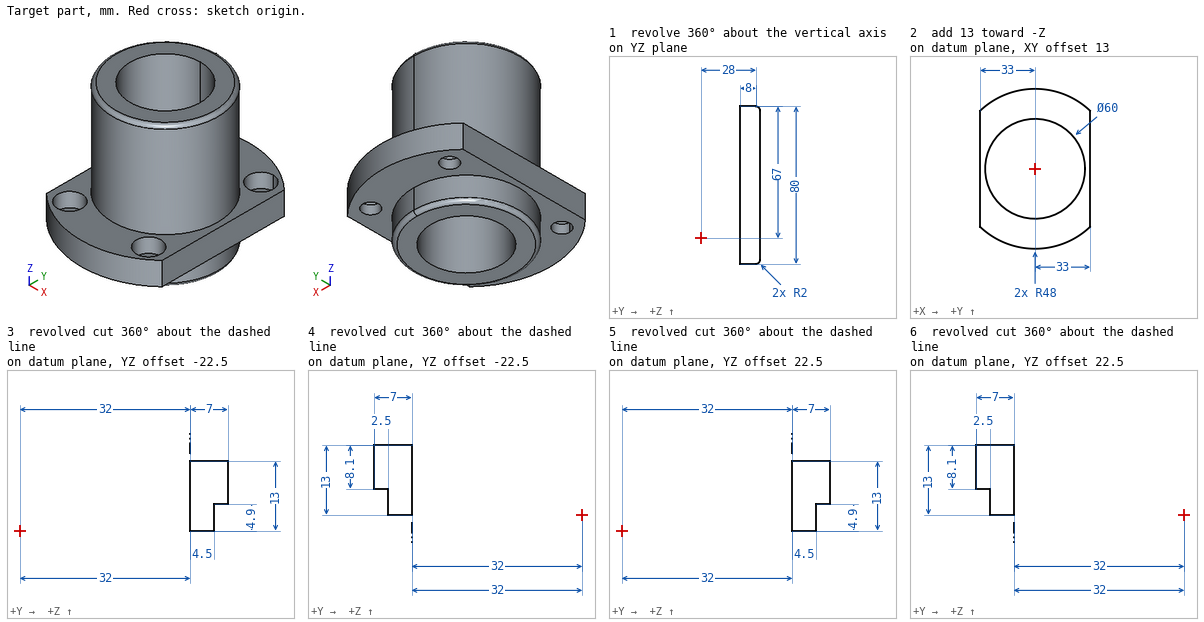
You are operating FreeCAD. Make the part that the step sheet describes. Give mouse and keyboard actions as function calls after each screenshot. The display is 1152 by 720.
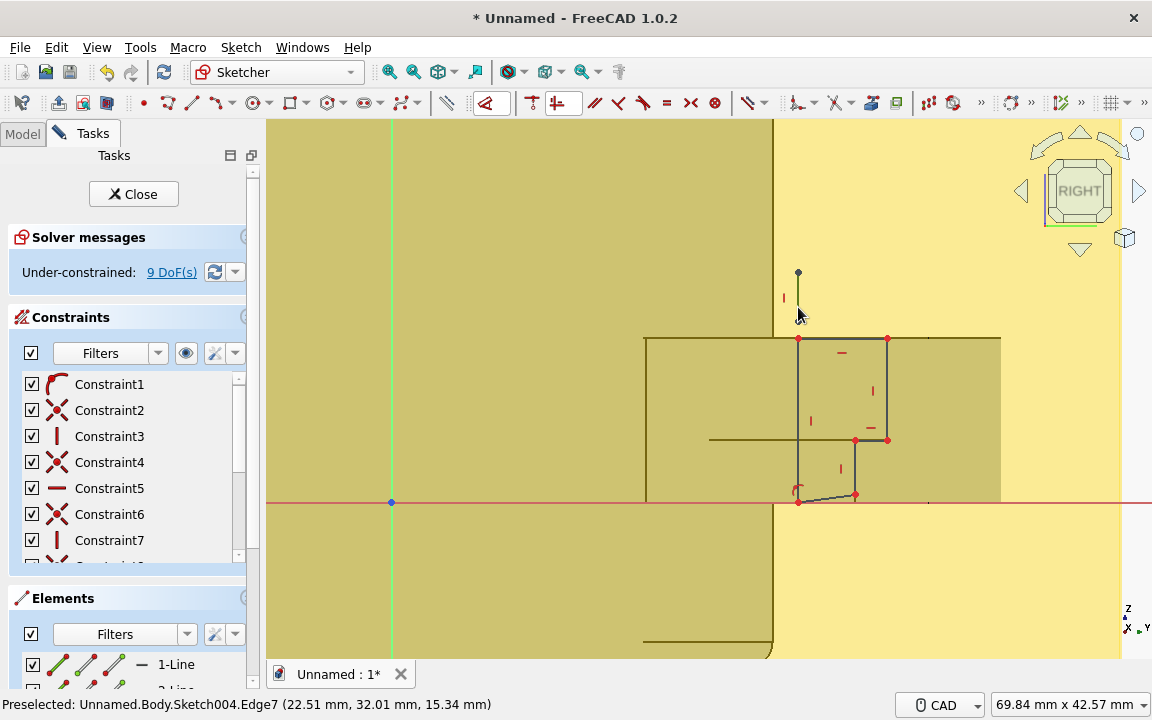
click(448, 104)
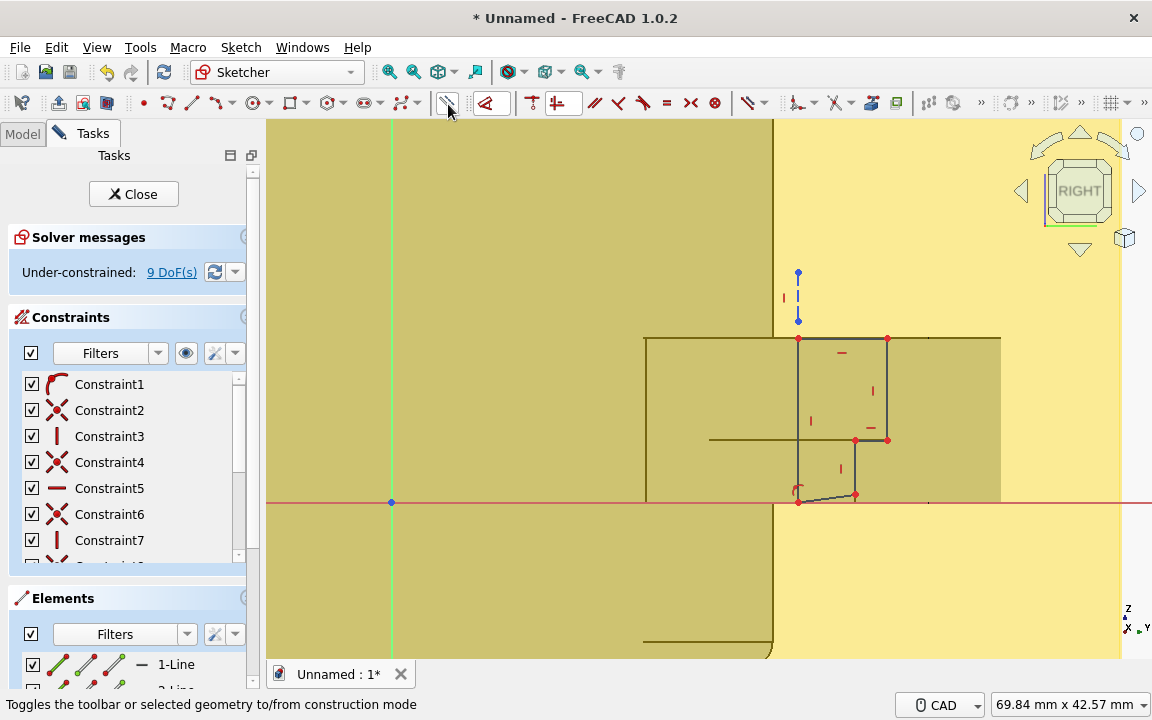
click(815, 500)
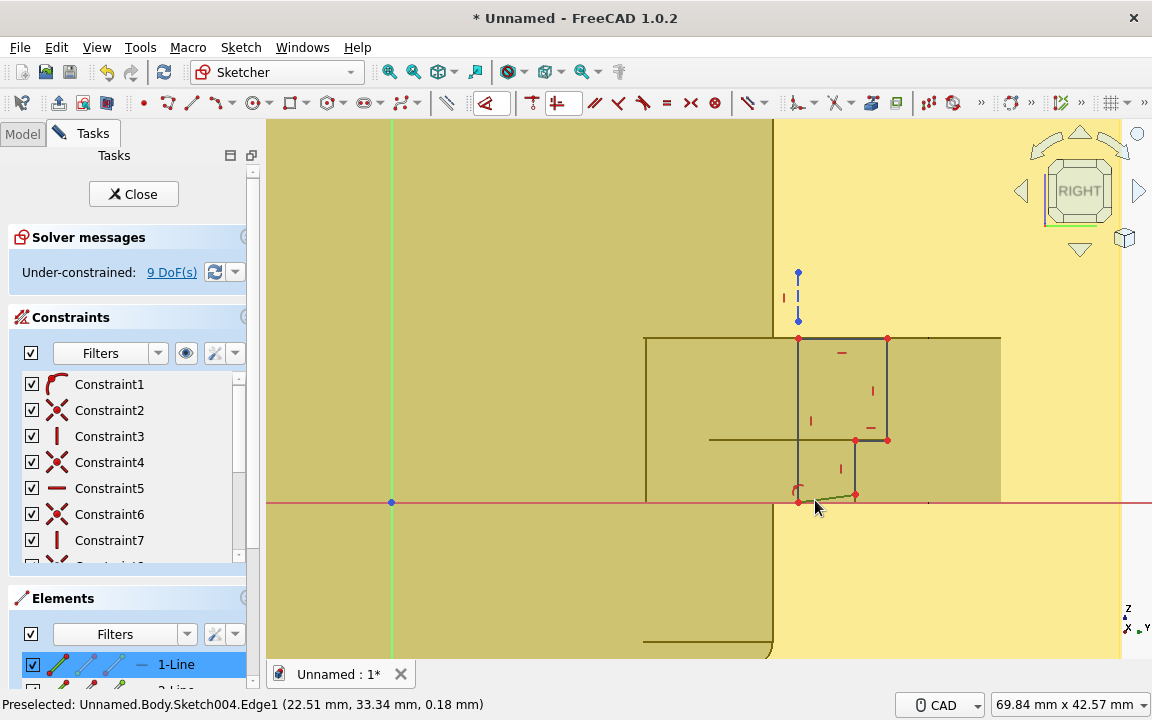
key(h)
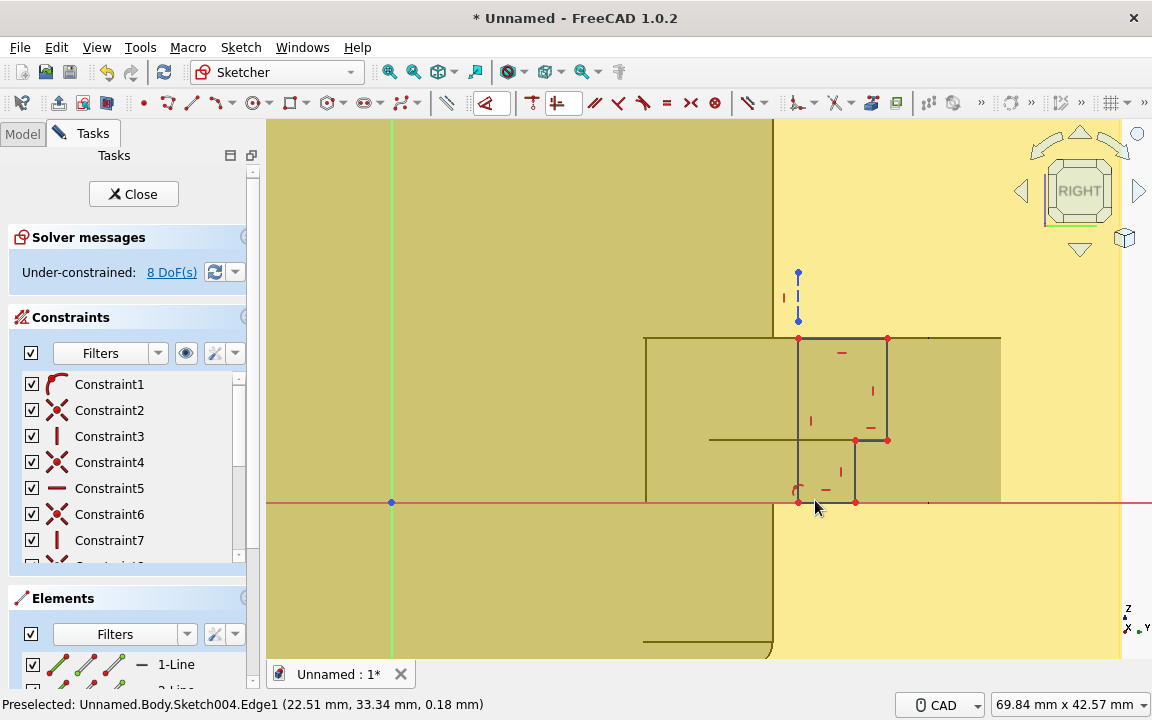
click(860, 339)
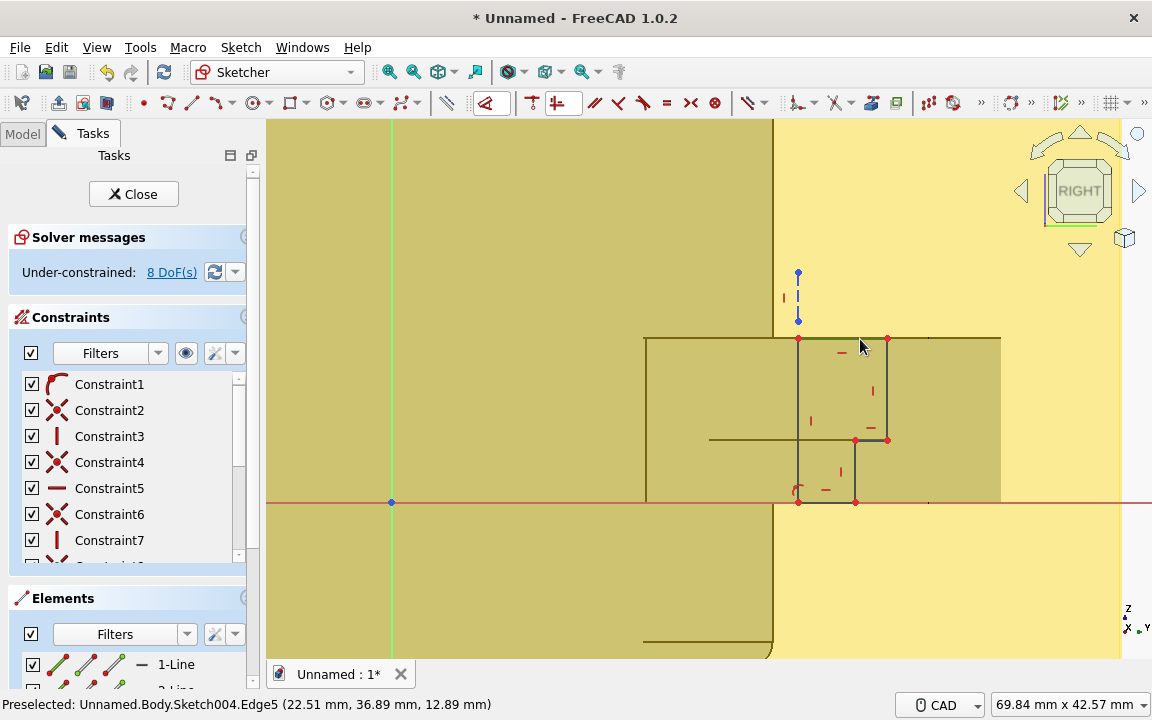
key(l)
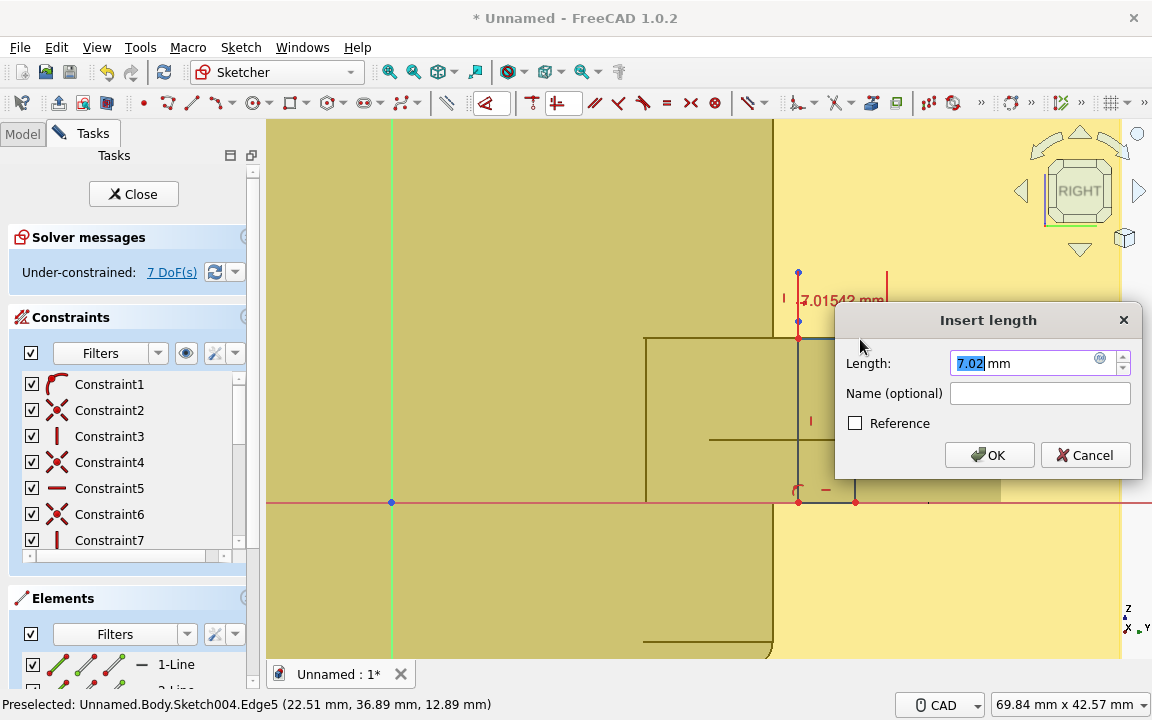
text(7)
key(Return)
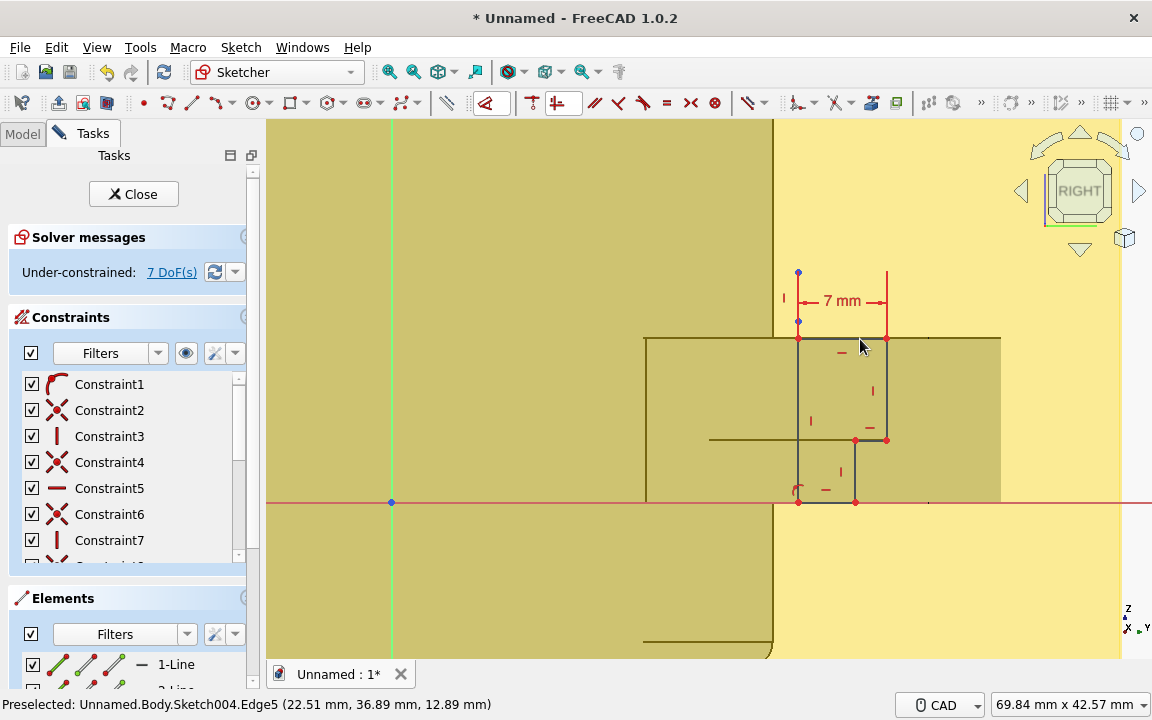
click(798, 388)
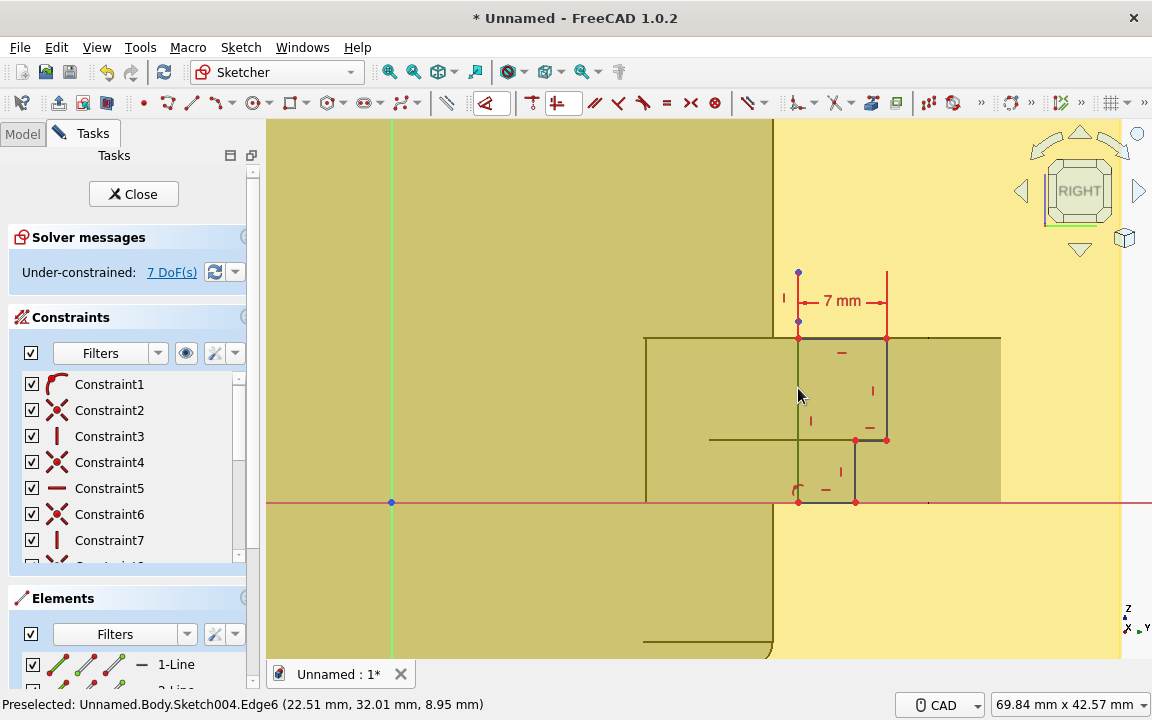
key(i)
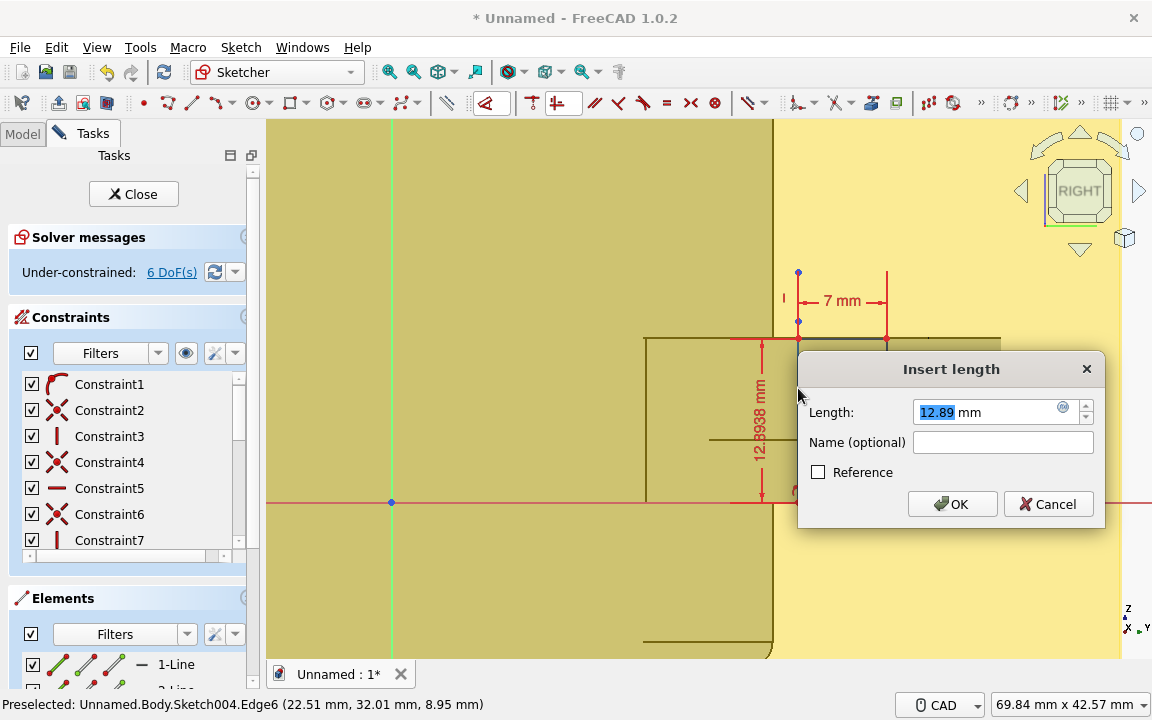
text(13)
key(Return)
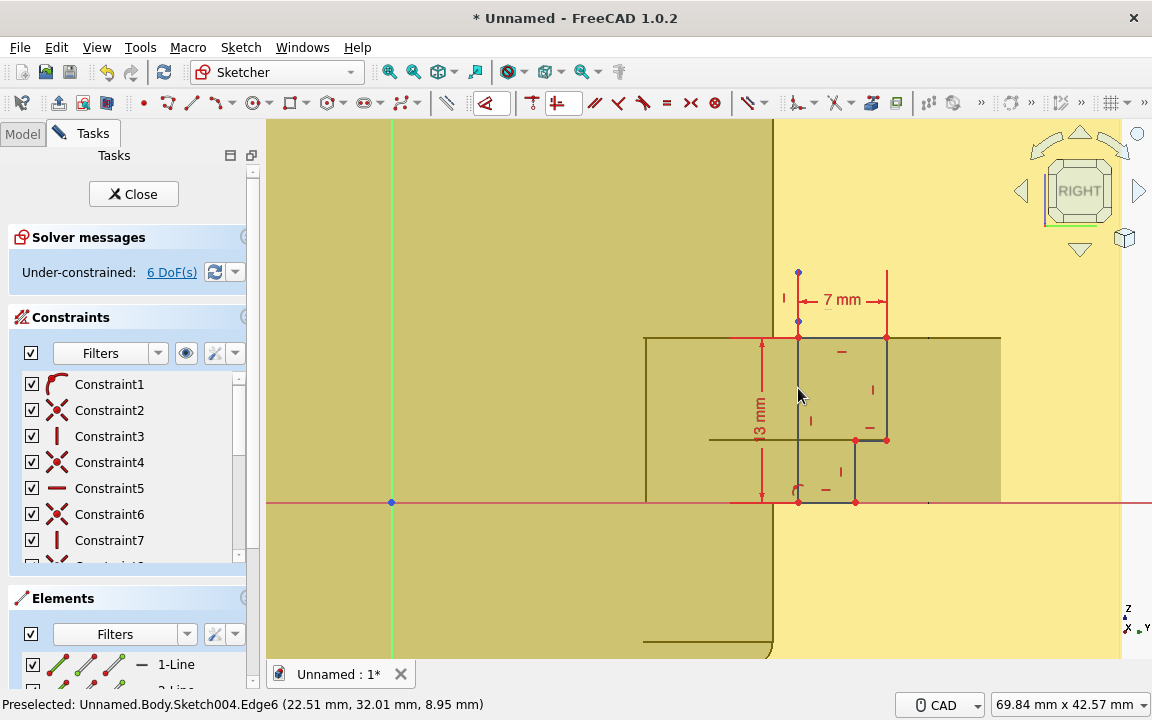
click(815, 503)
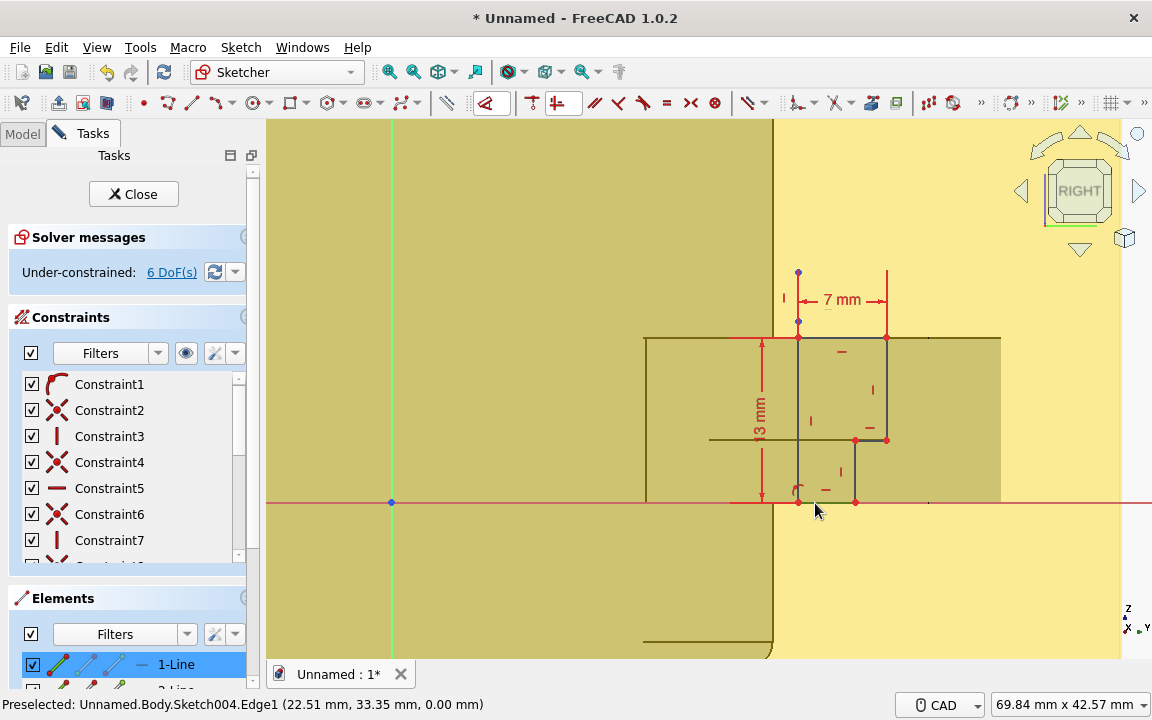
key(l)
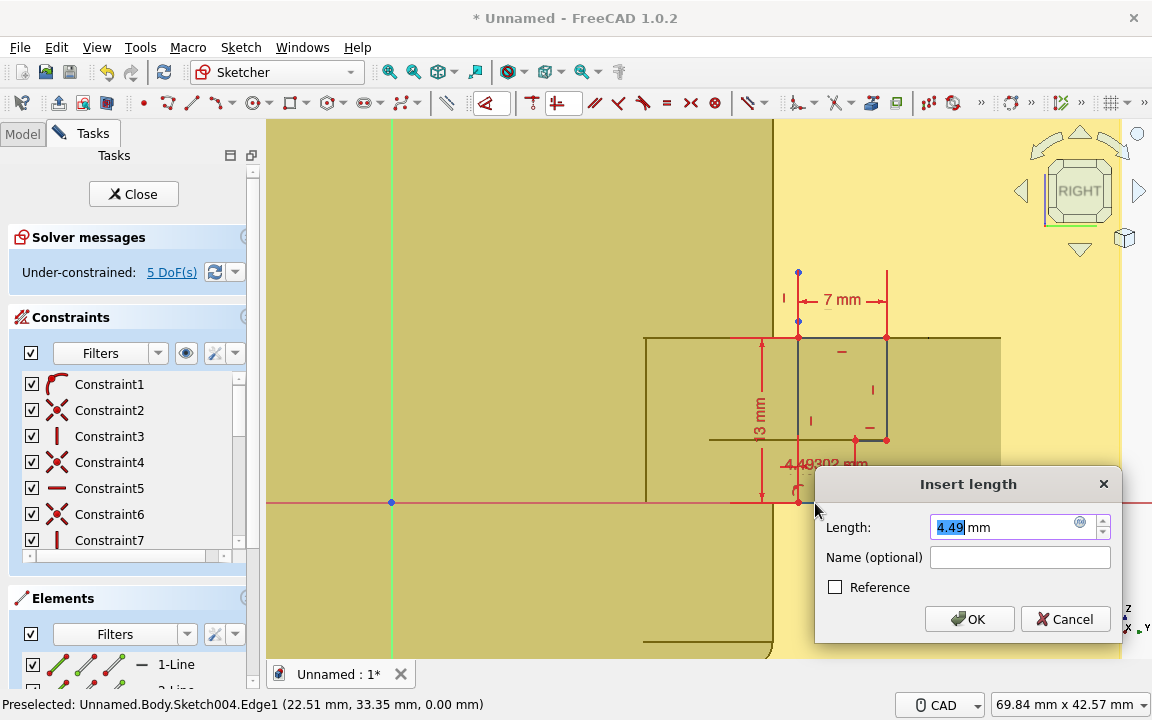
text(4.5)
key(Return)